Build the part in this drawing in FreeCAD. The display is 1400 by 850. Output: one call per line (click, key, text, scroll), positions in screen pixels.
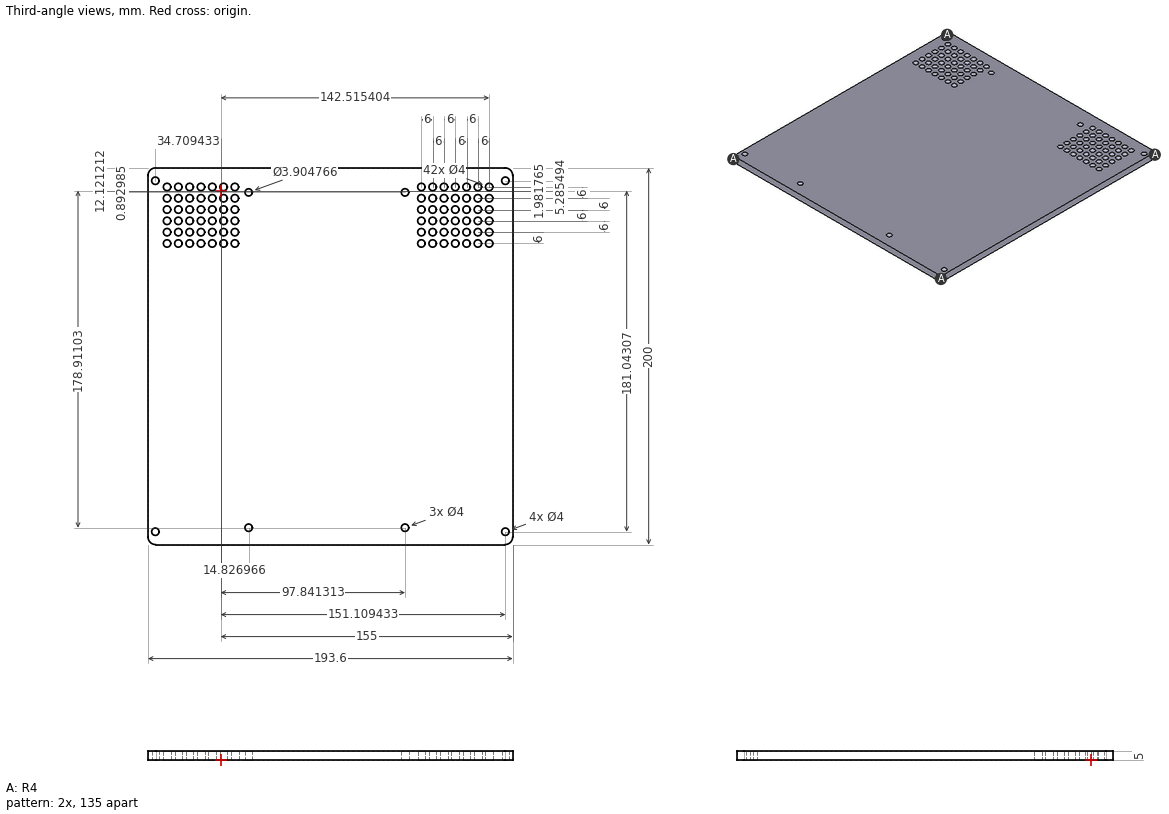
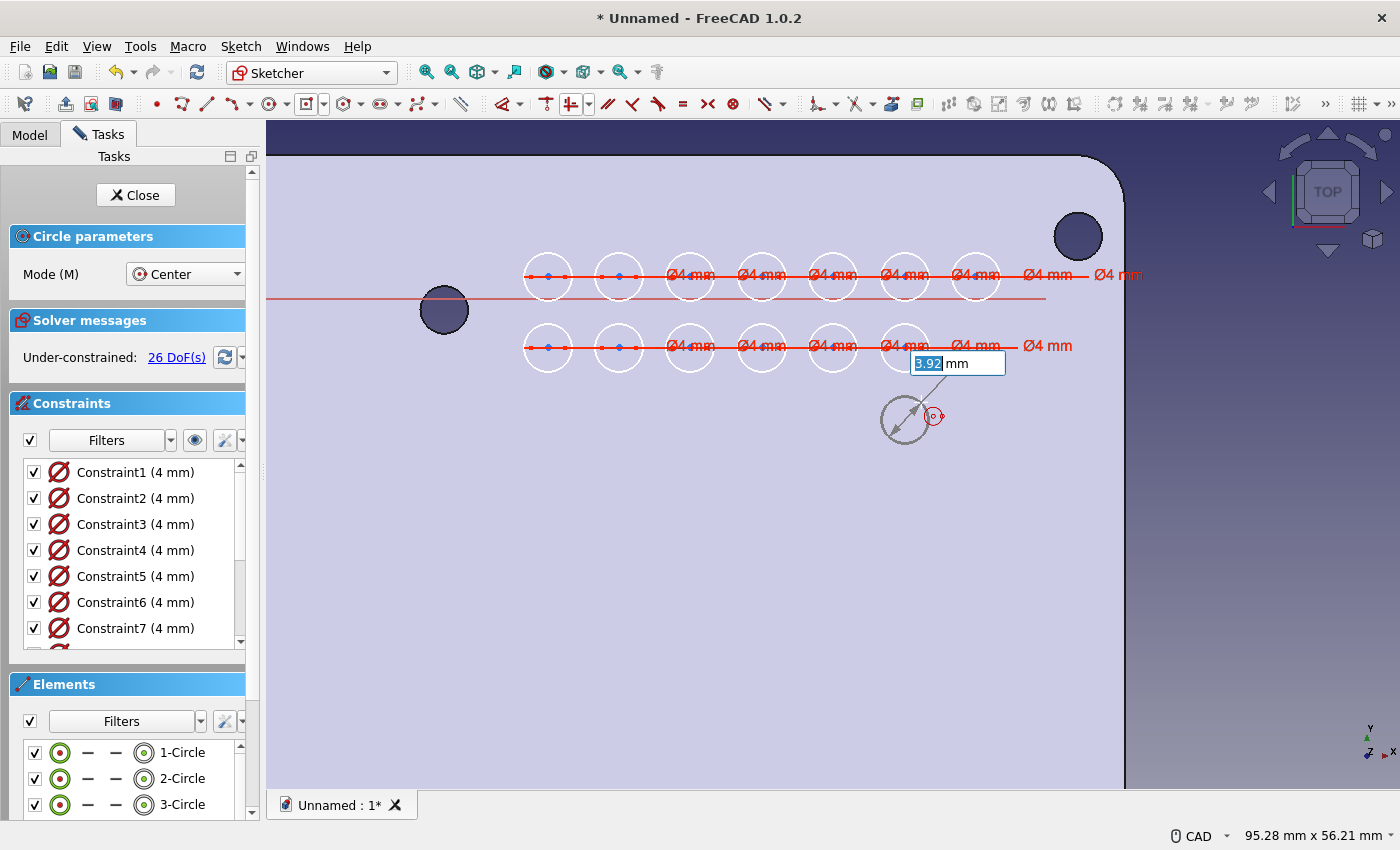
text(4)
key(Return)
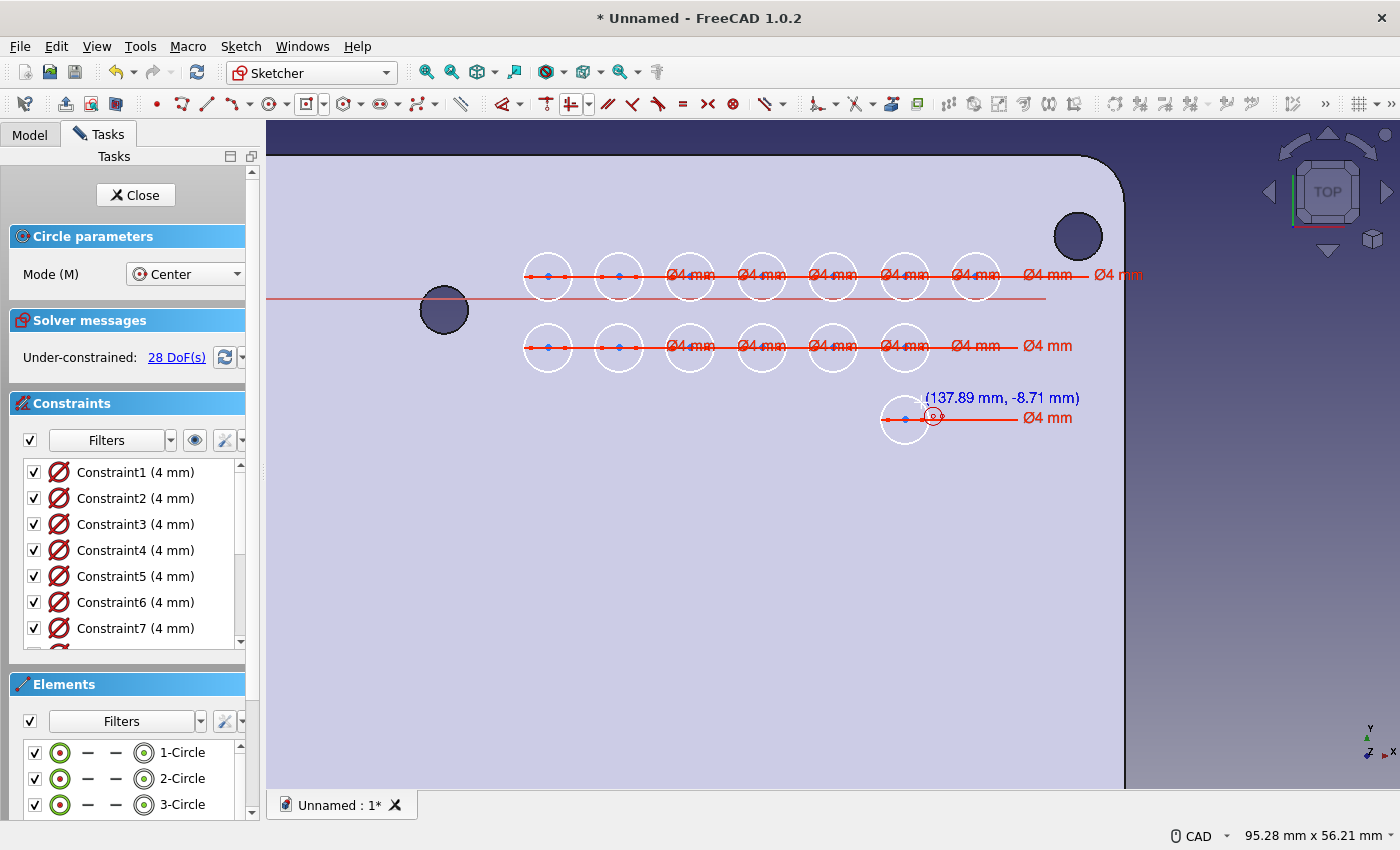
click(833, 419)
move(850, 402)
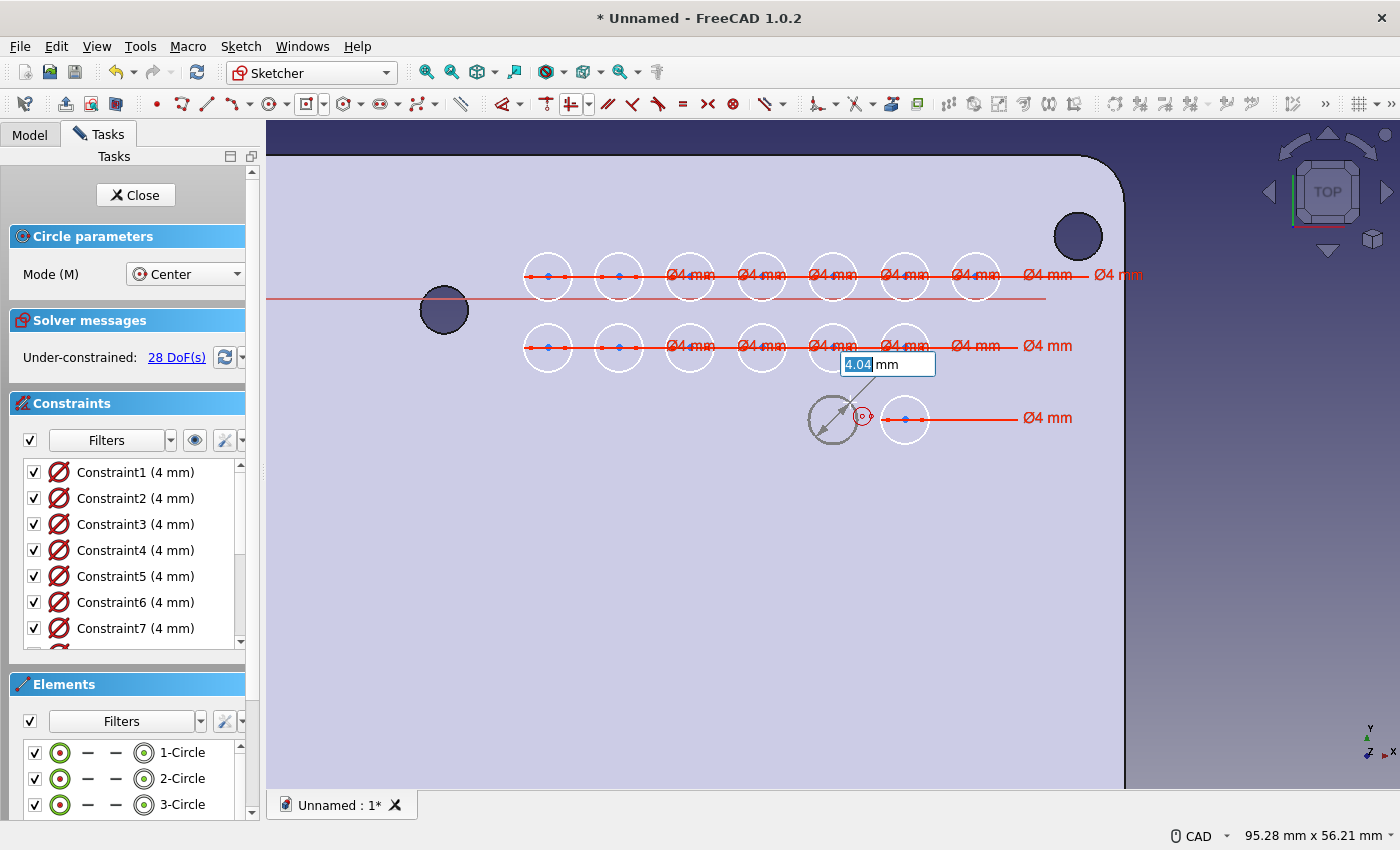
text(4)
key(Return)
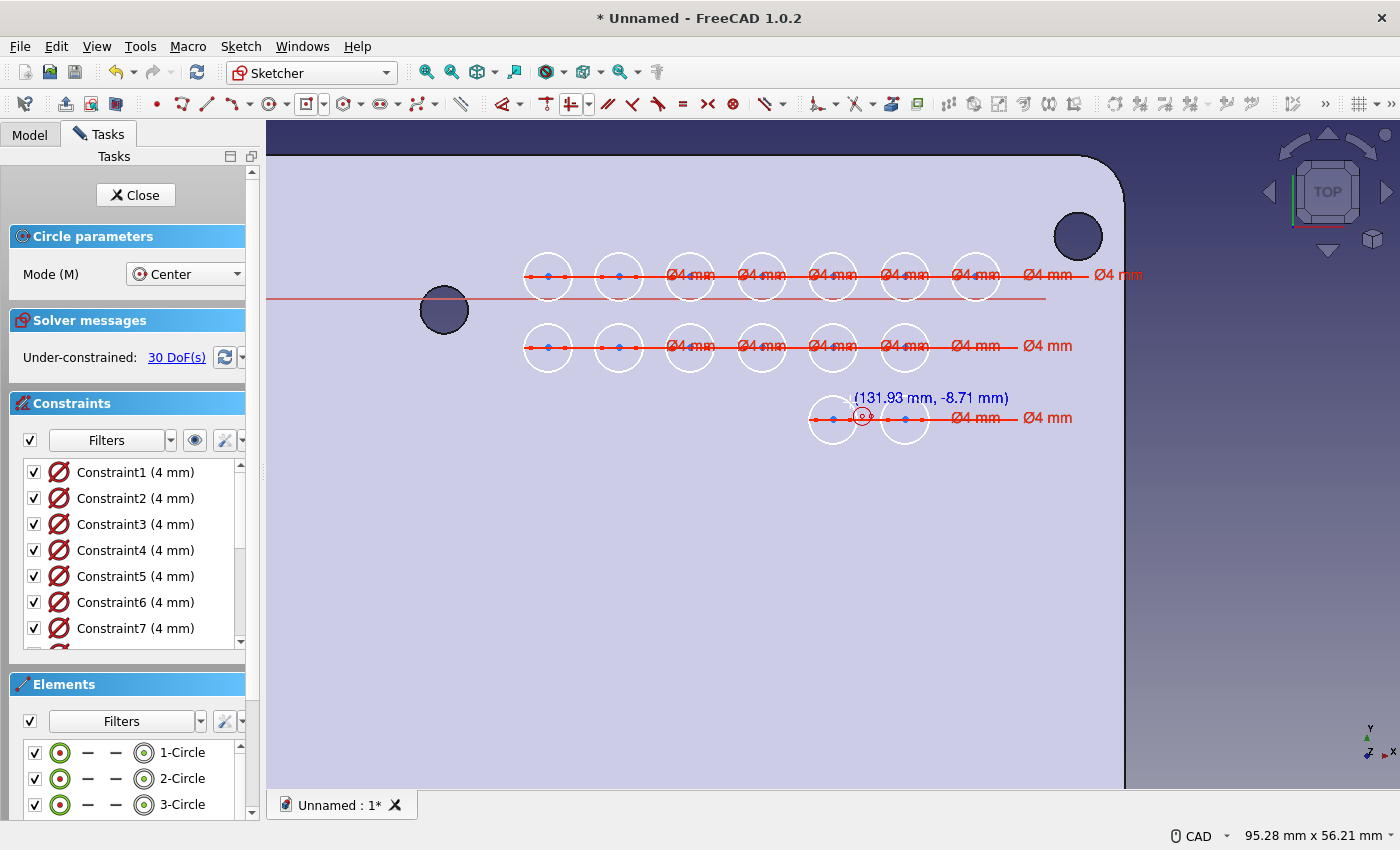
click(762, 419)
move(779, 402)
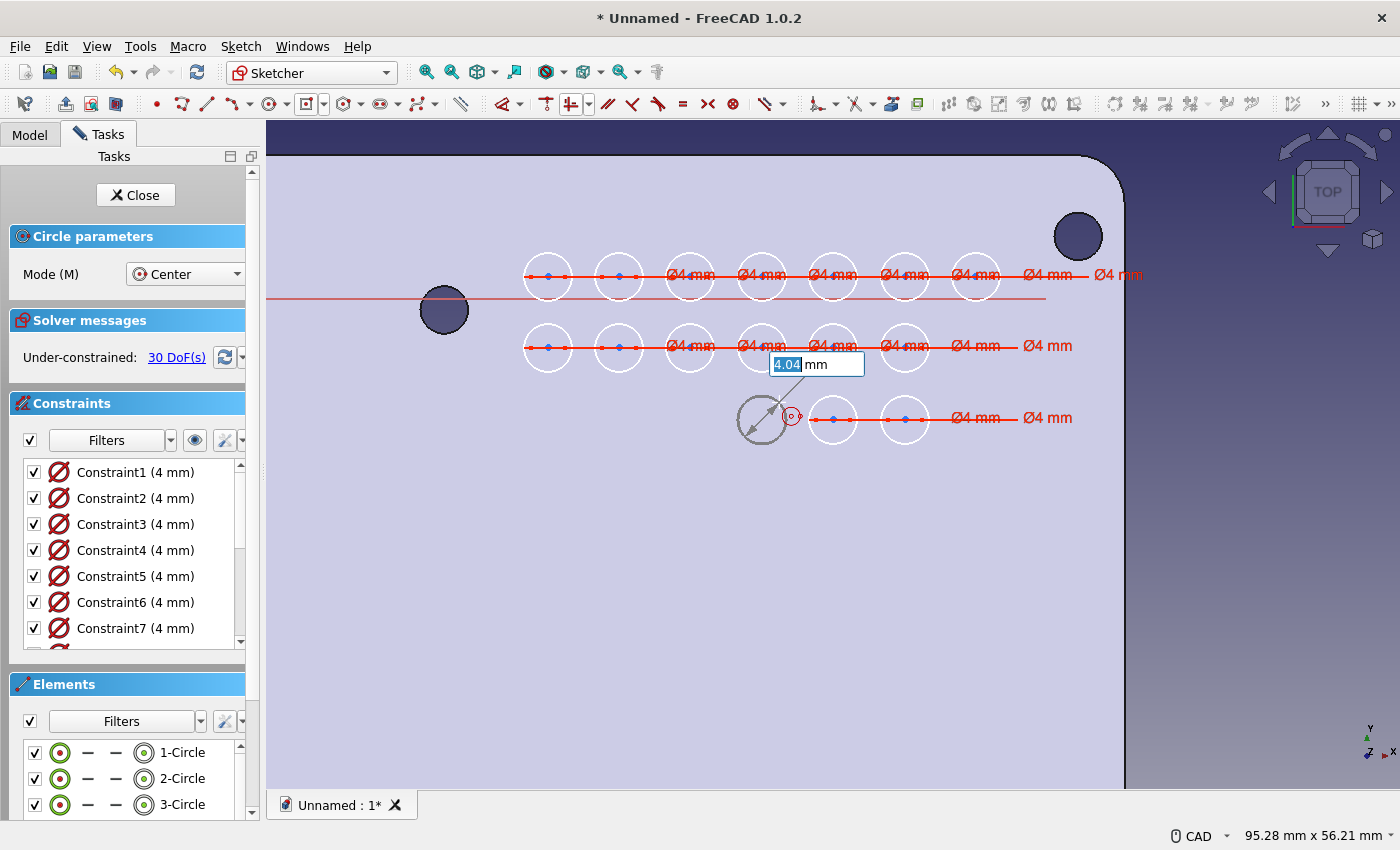
text(4)
key(Return)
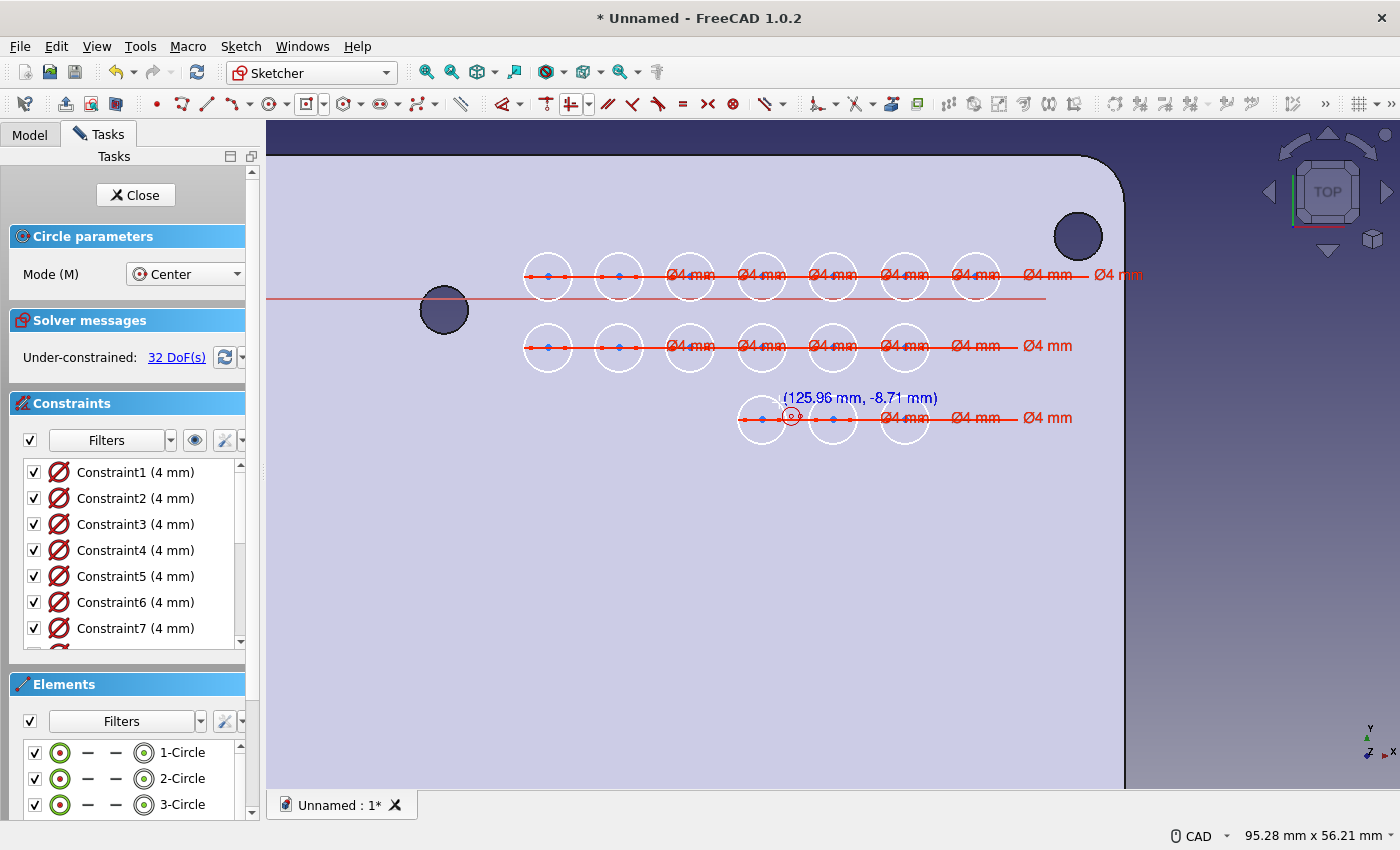
click(690, 419)
move(707, 402)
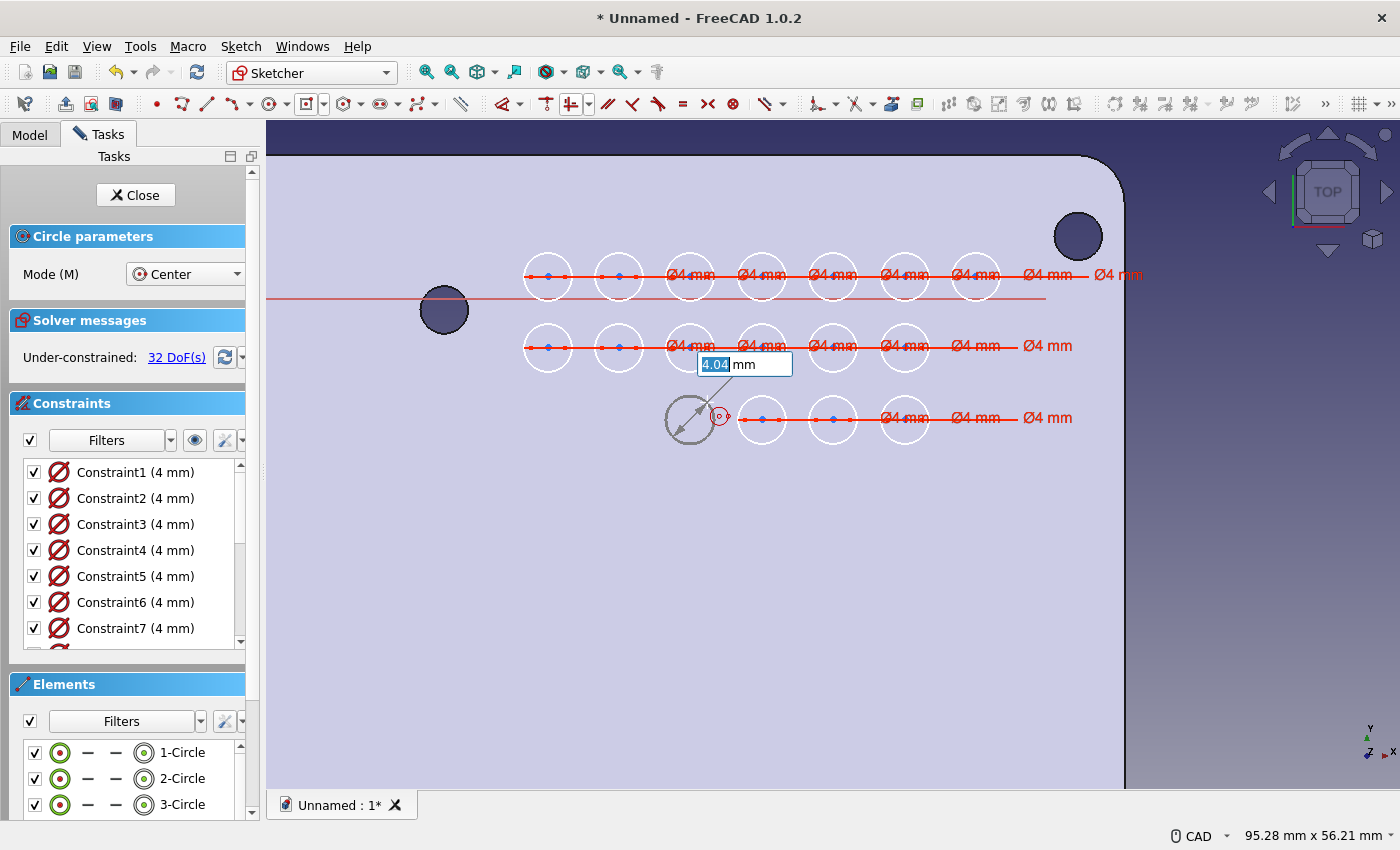
text(4)
key(Return)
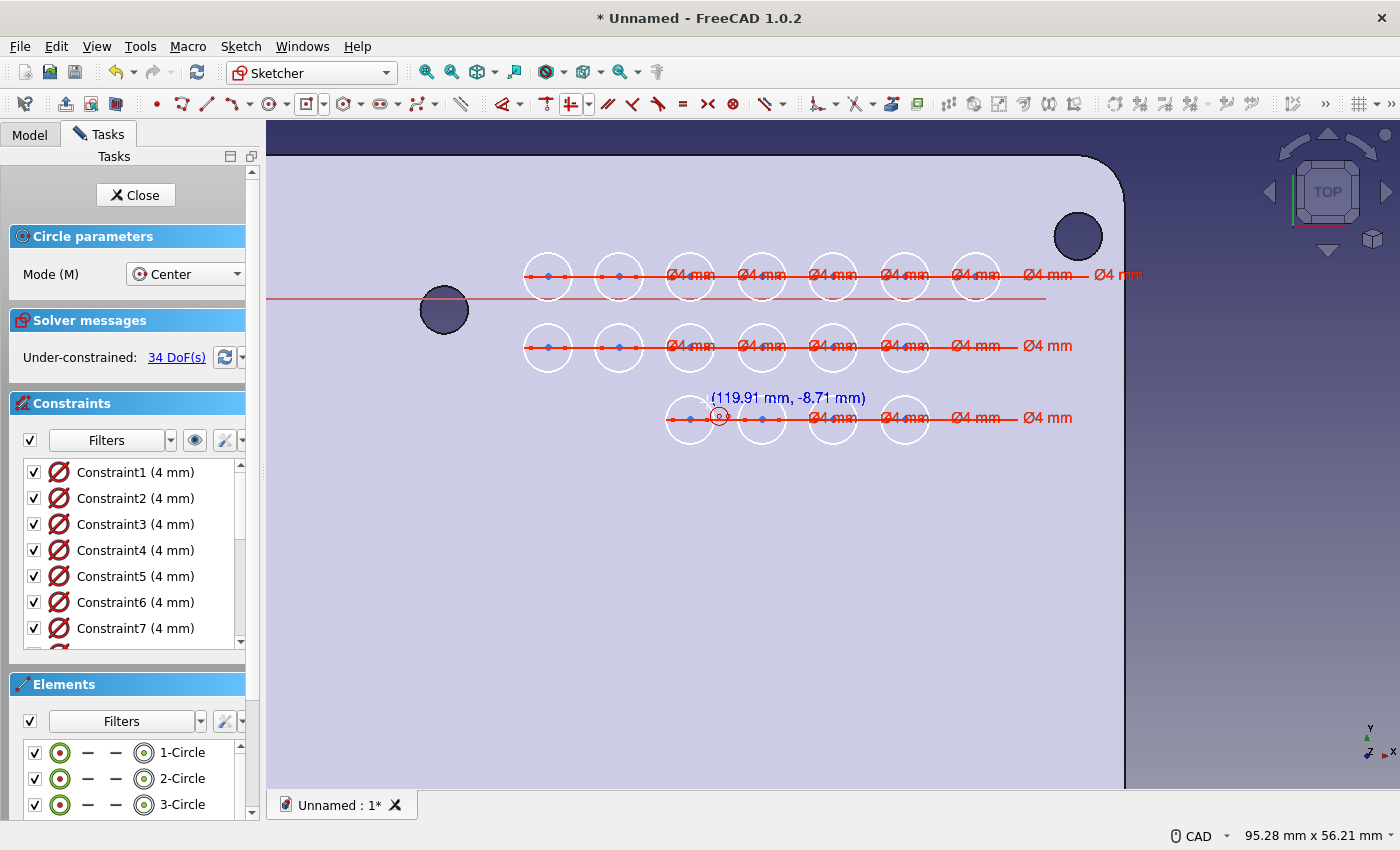
click(619, 419)
move(636, 402)